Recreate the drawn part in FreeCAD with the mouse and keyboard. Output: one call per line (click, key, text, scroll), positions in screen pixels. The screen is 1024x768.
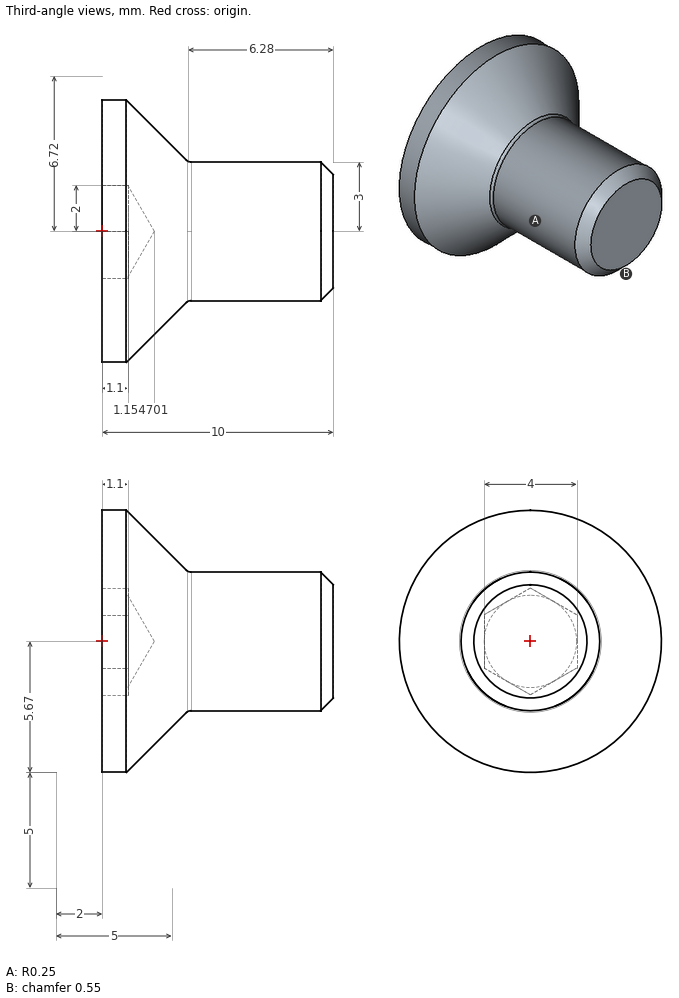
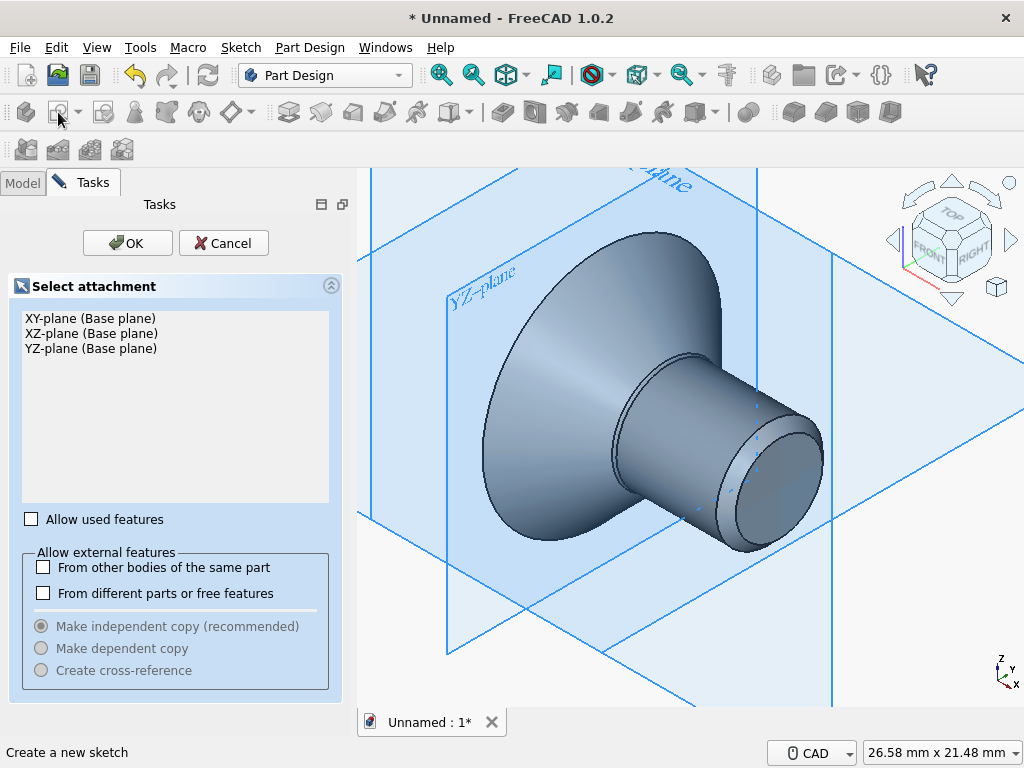
click(82, 334)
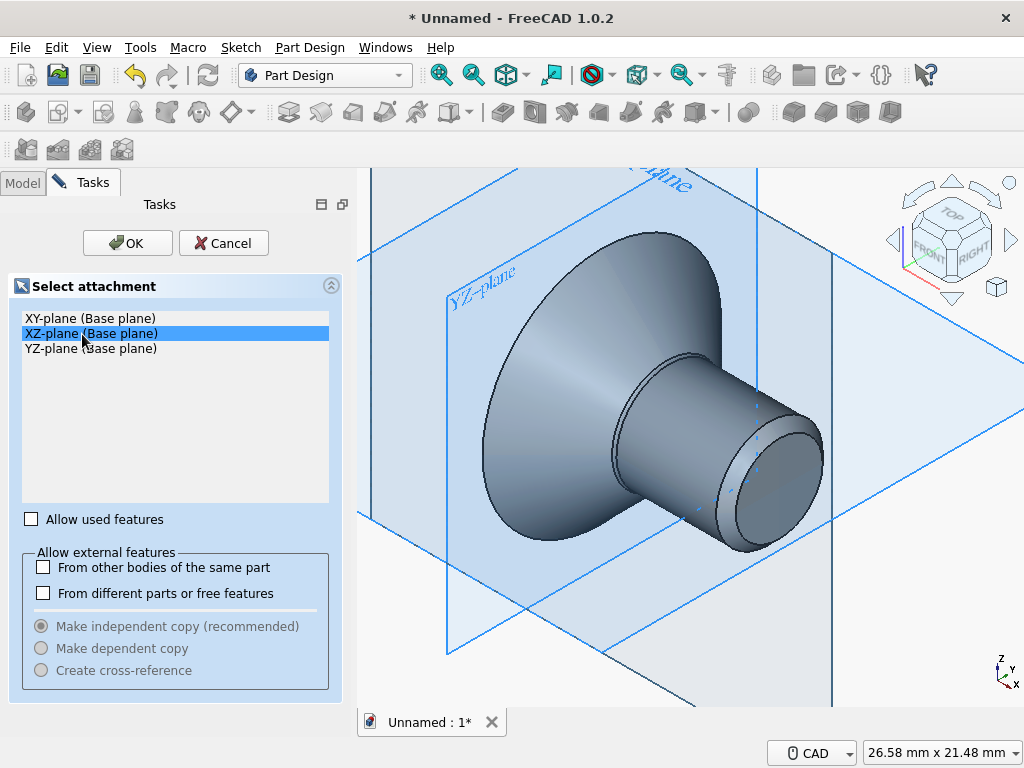
click(128, 243)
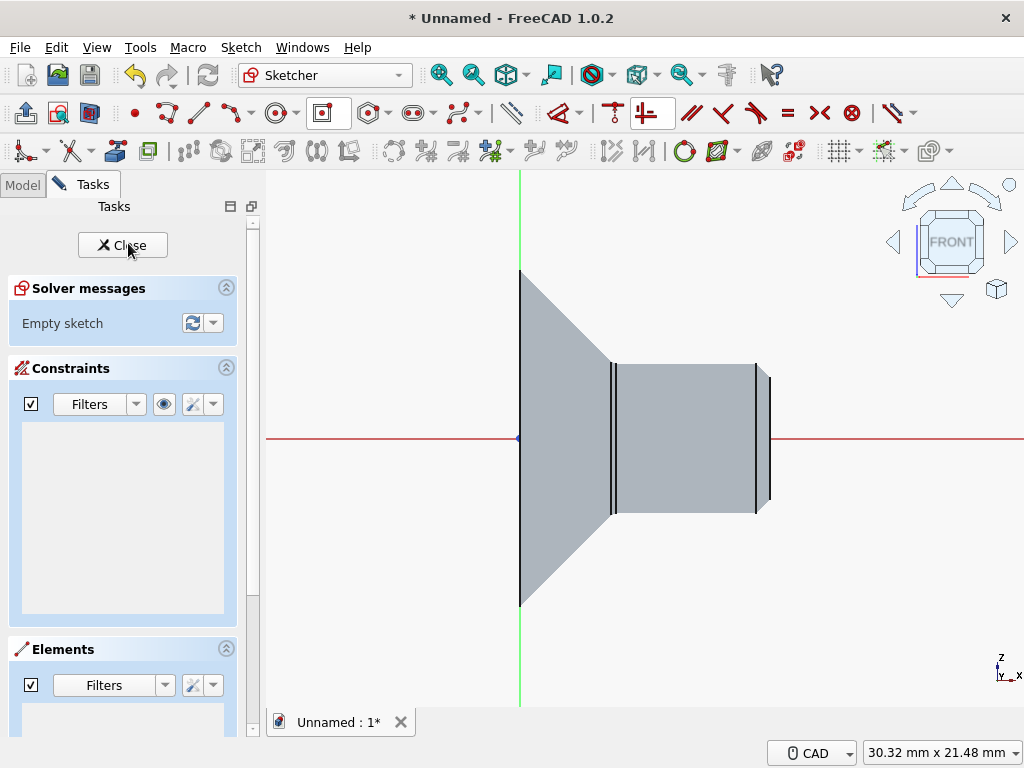
key(q)
key(s)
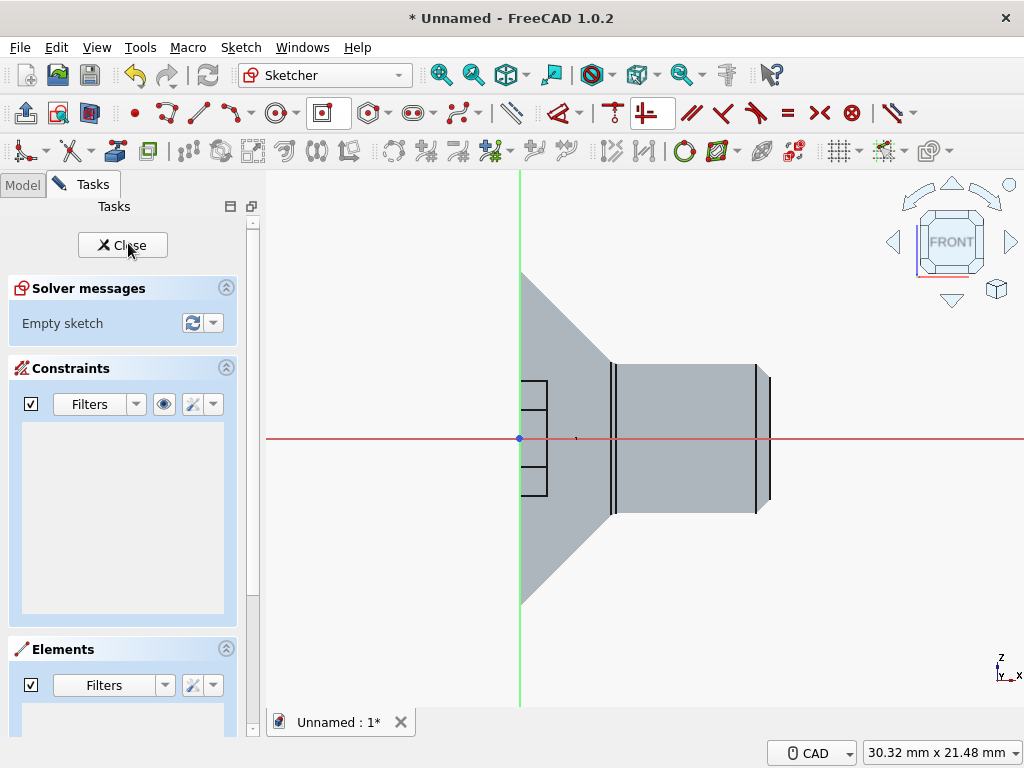
scroll(775, 198, down, 1)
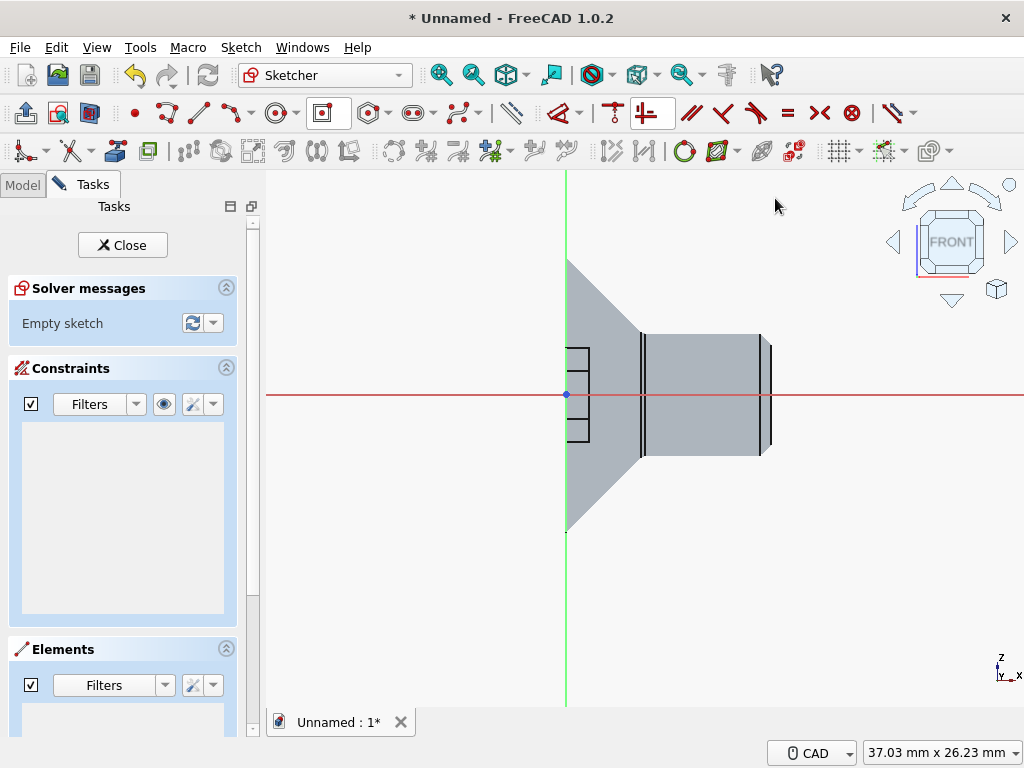
scroll(577, 638, up, 2)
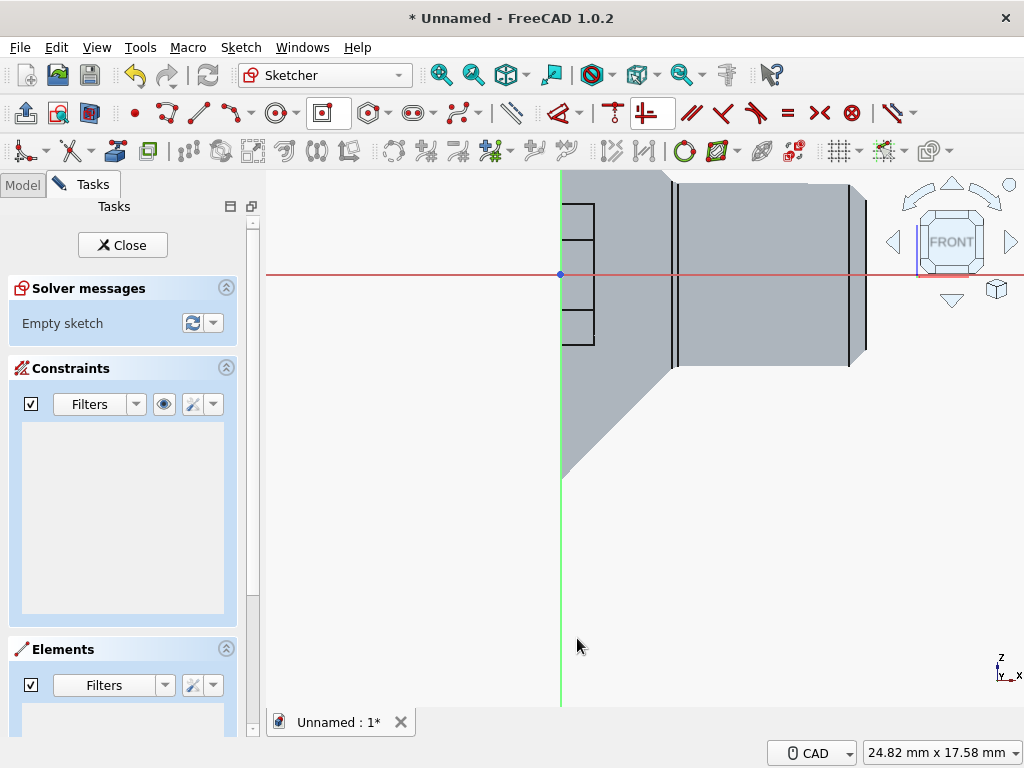
key(g)
key(r)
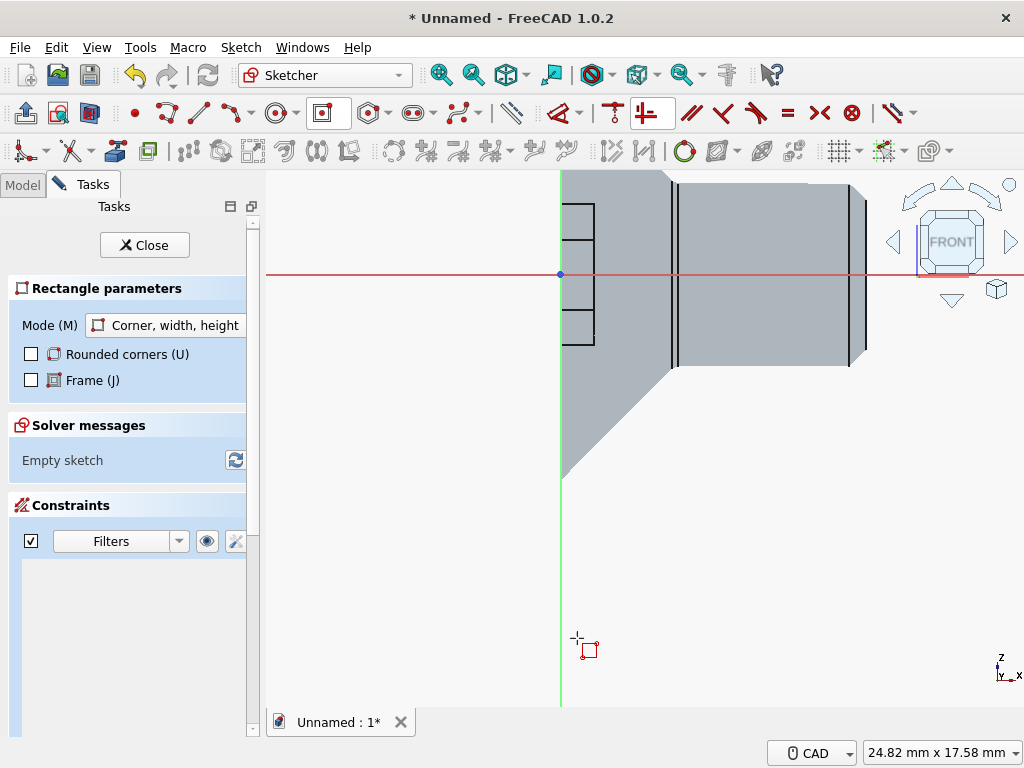
click(500, 448)
click(653, 601)
key(Escape)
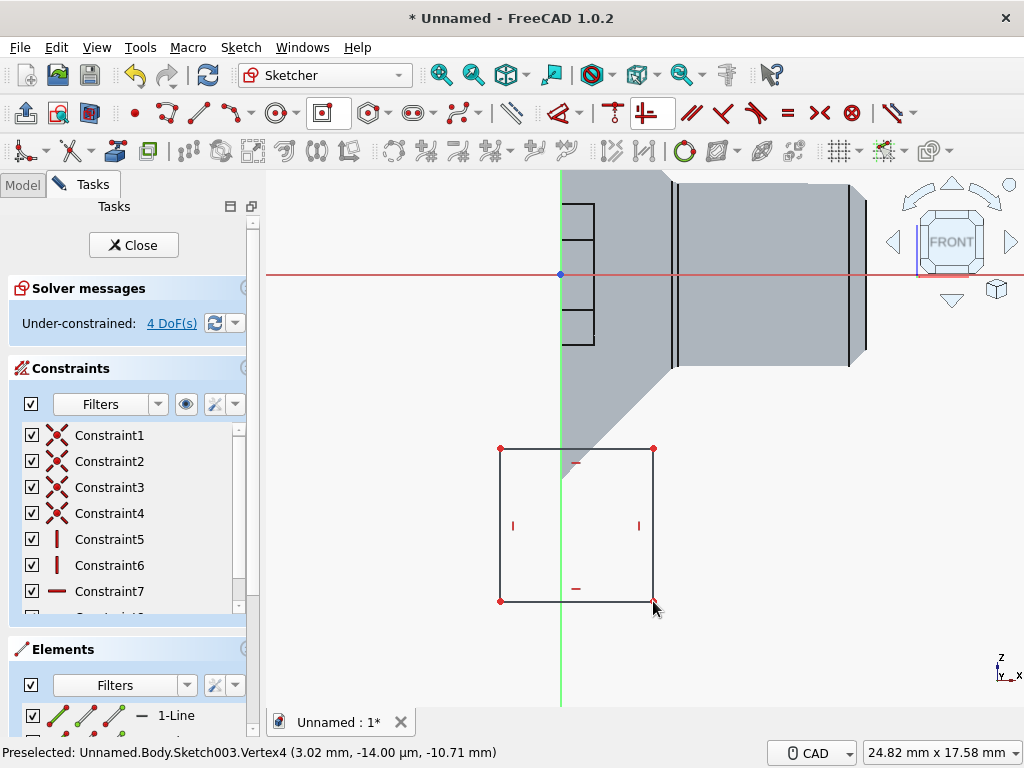
key(d)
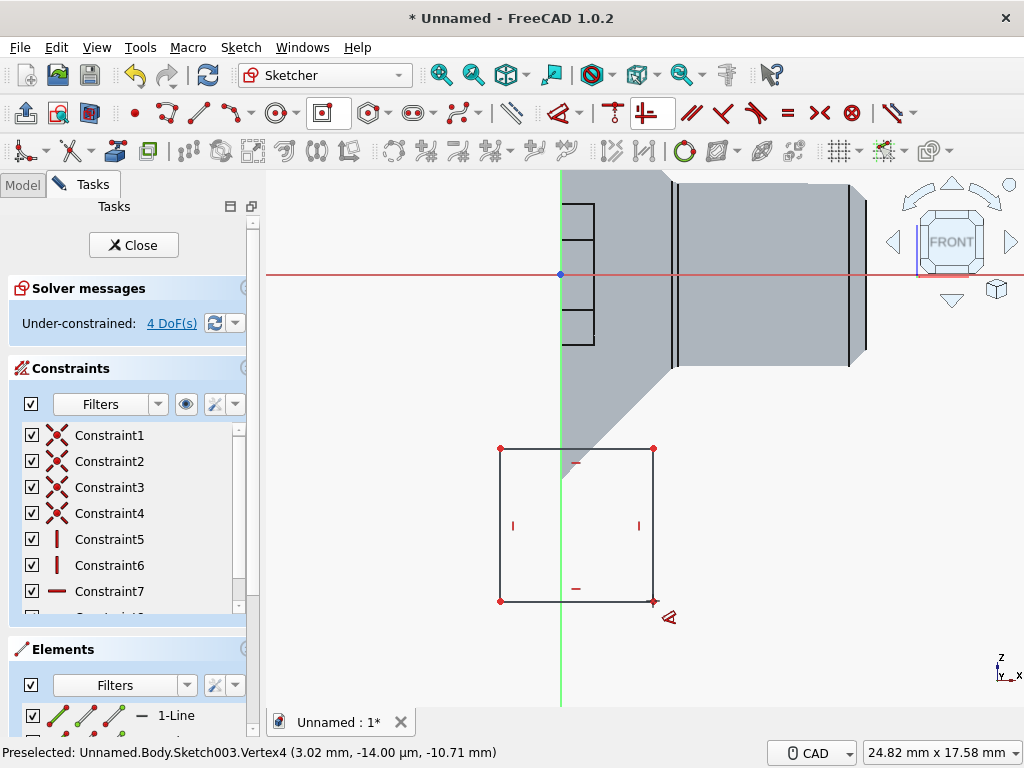
click(500, 495)
click(466, 525)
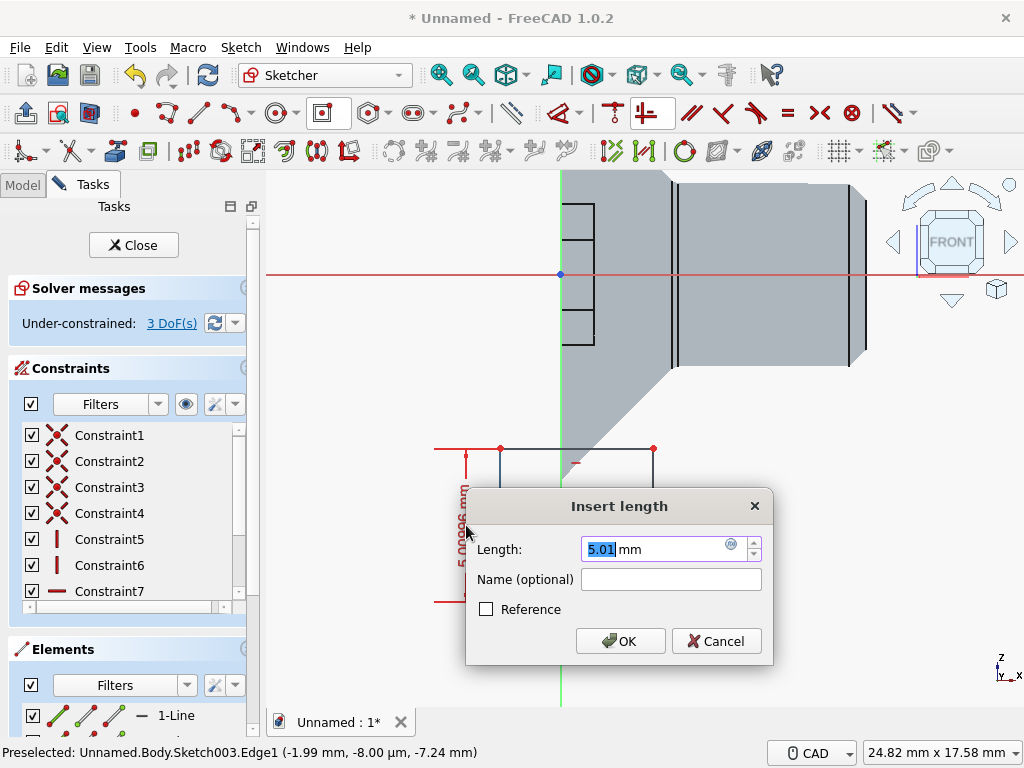
text(5)
key(Return)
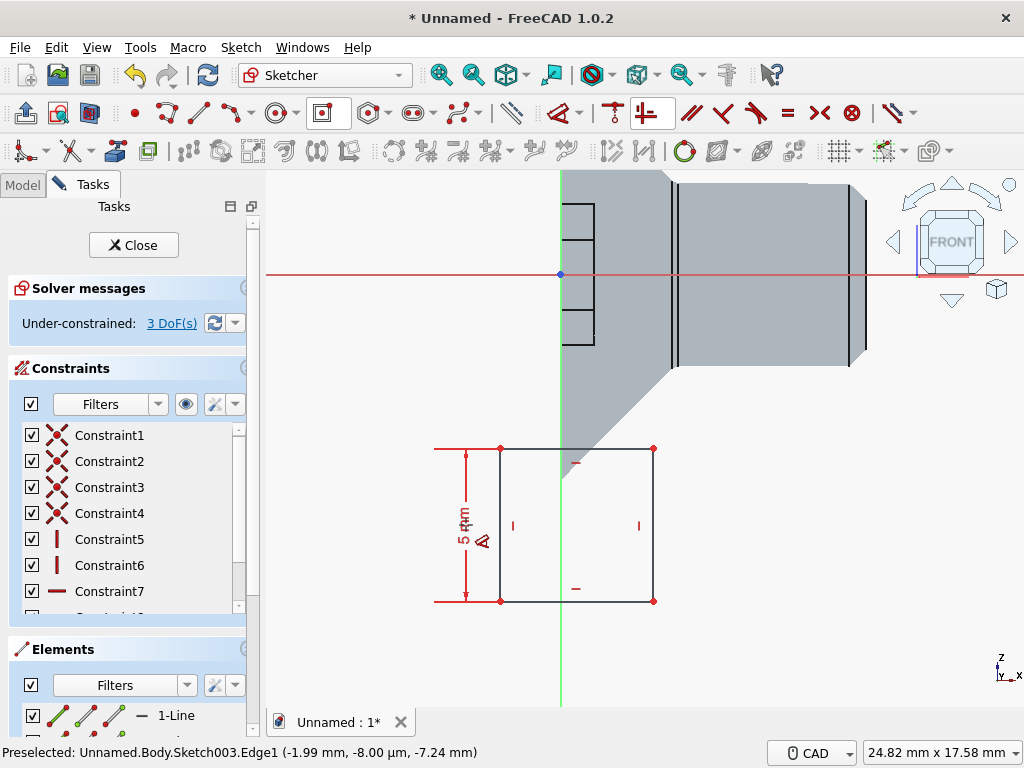
click(546, 602)
click(576, 636)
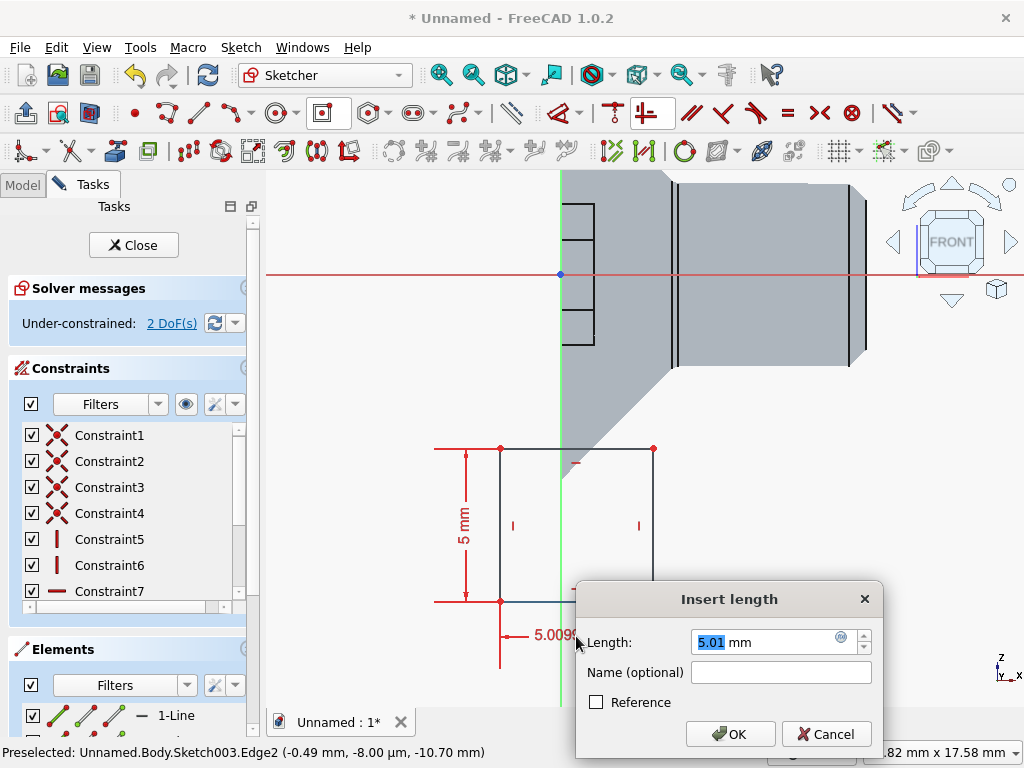
text(5)
key(Return)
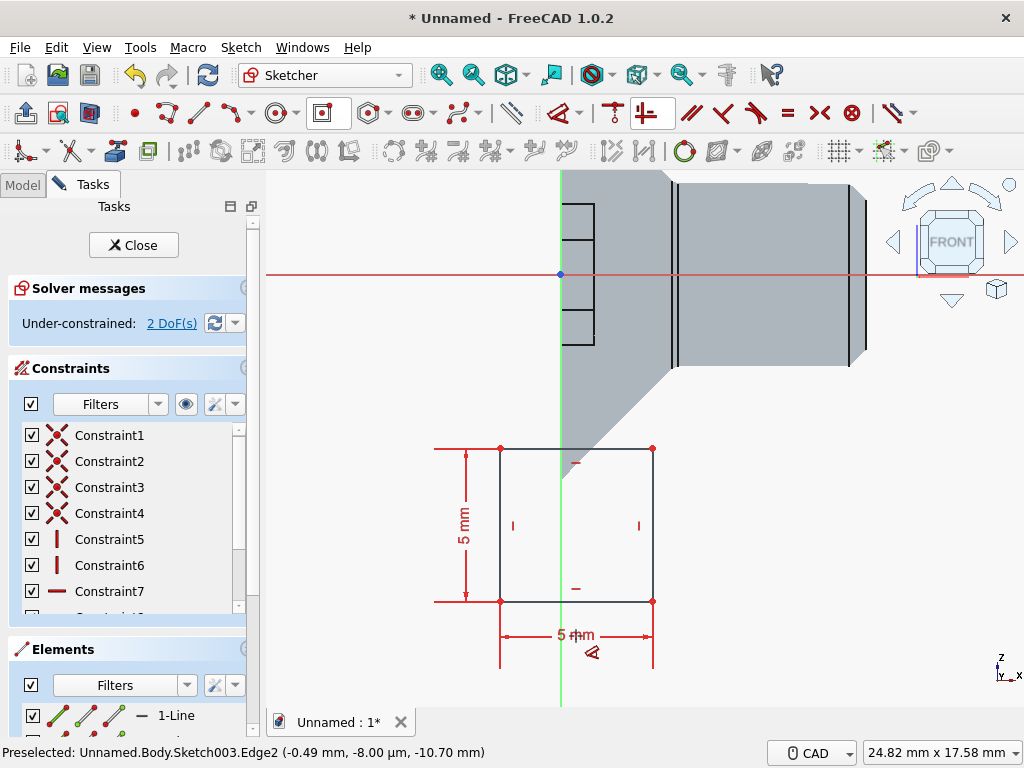
click(500, 449)
click(530, 241)